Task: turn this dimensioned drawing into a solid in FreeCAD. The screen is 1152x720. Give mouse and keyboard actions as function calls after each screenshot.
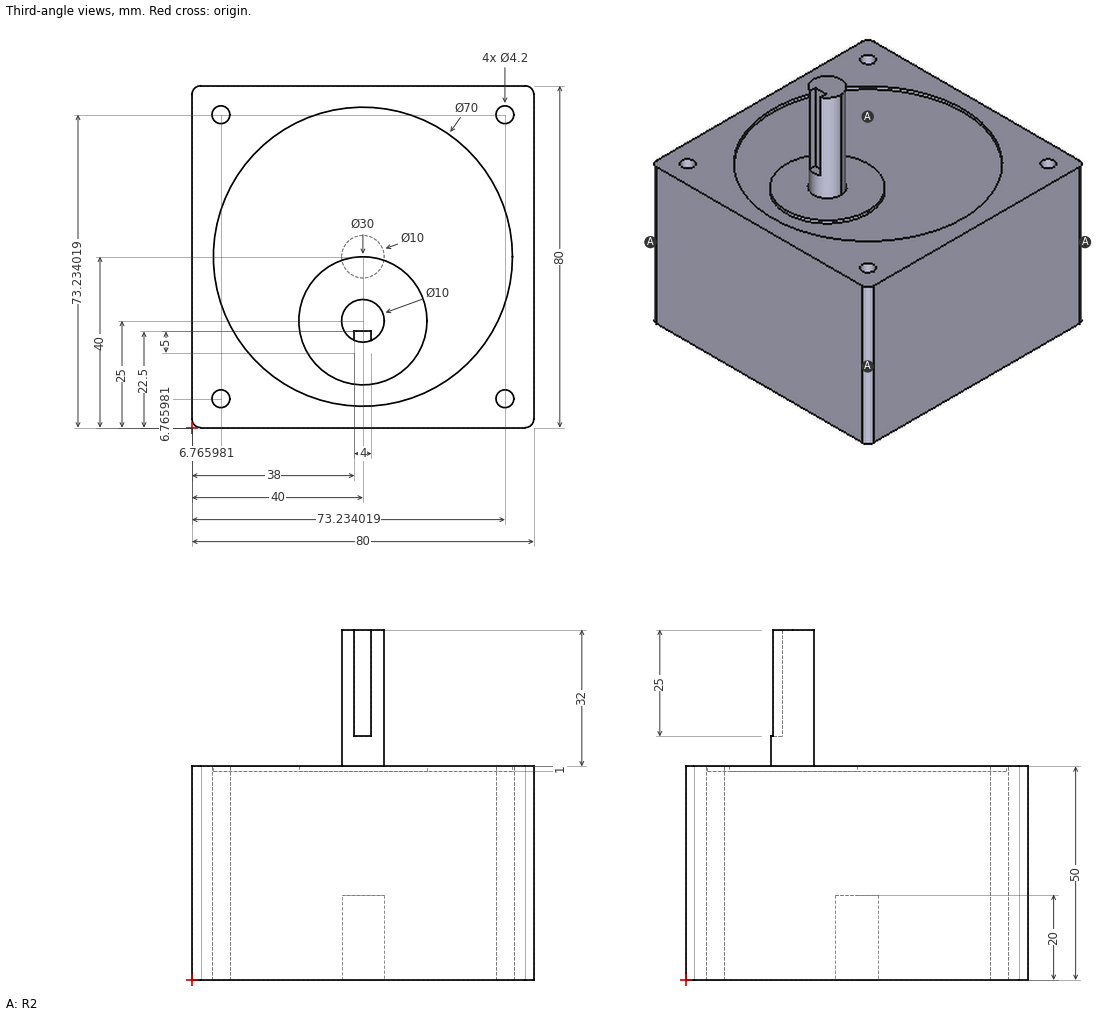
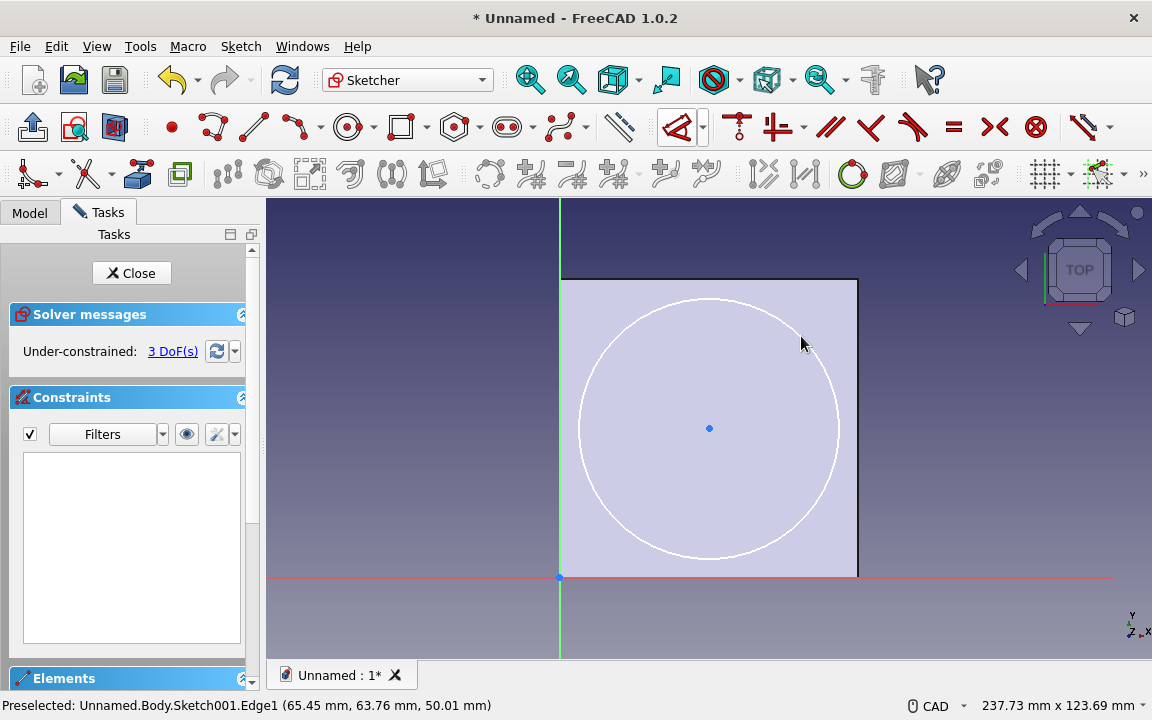
click(801, 337)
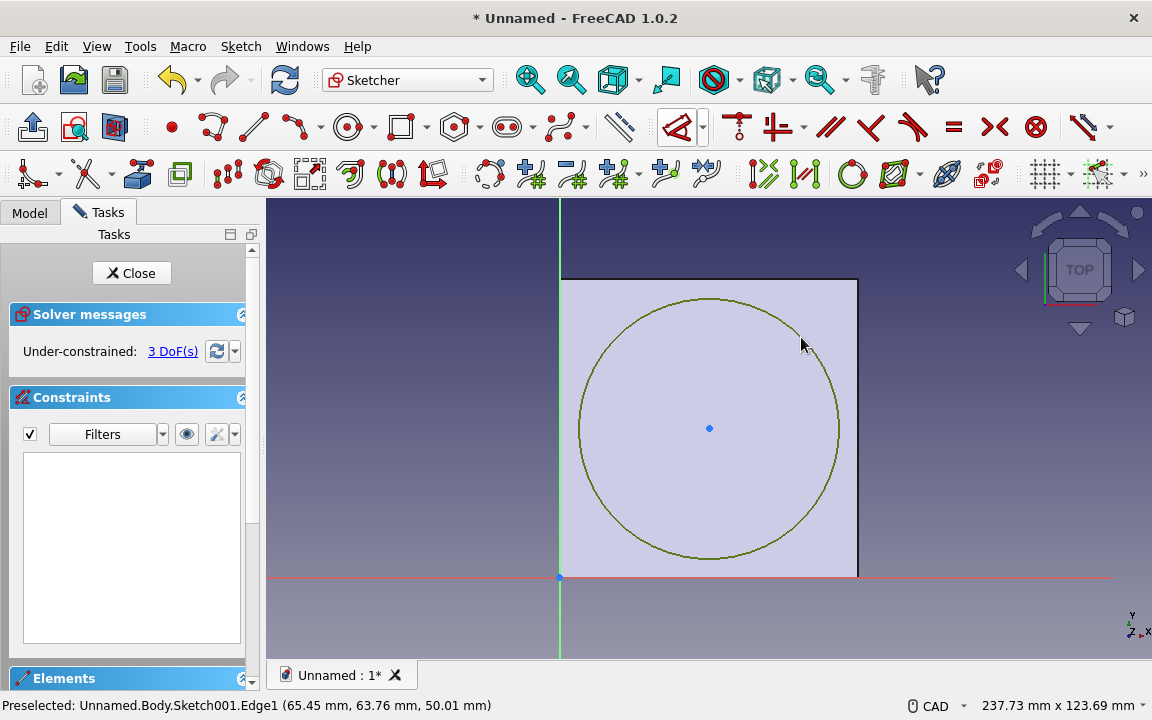
key(k)
key(o)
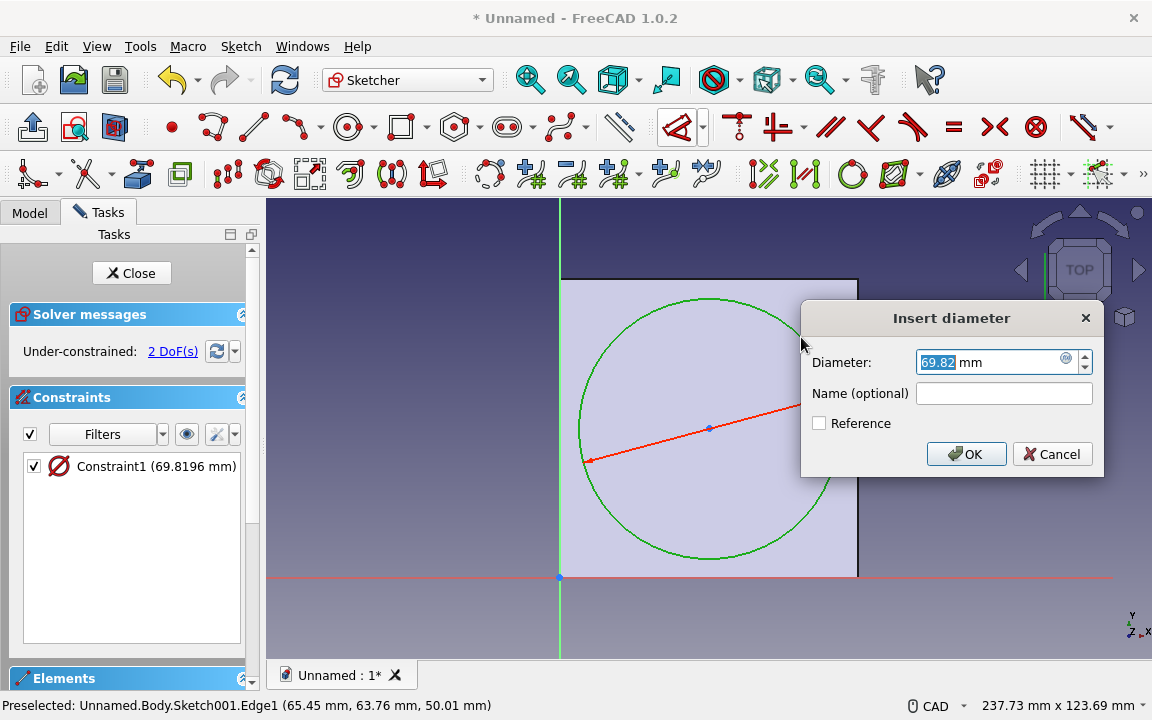
text(70)
key(Return)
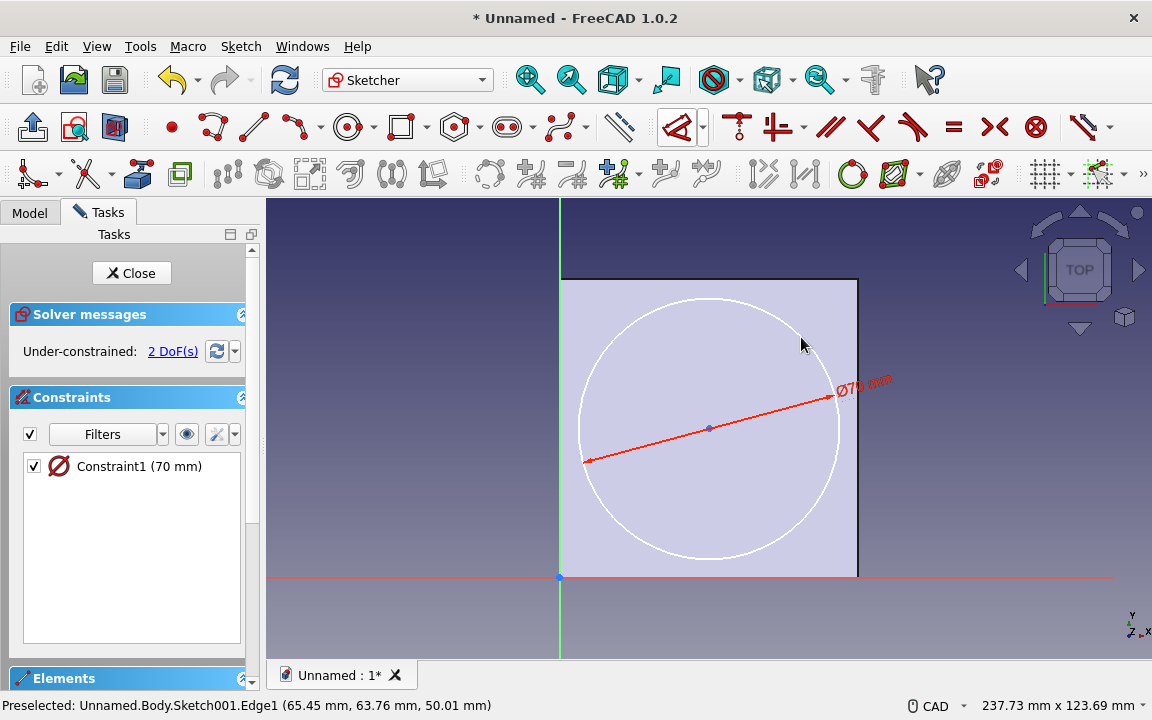
click(709, 429)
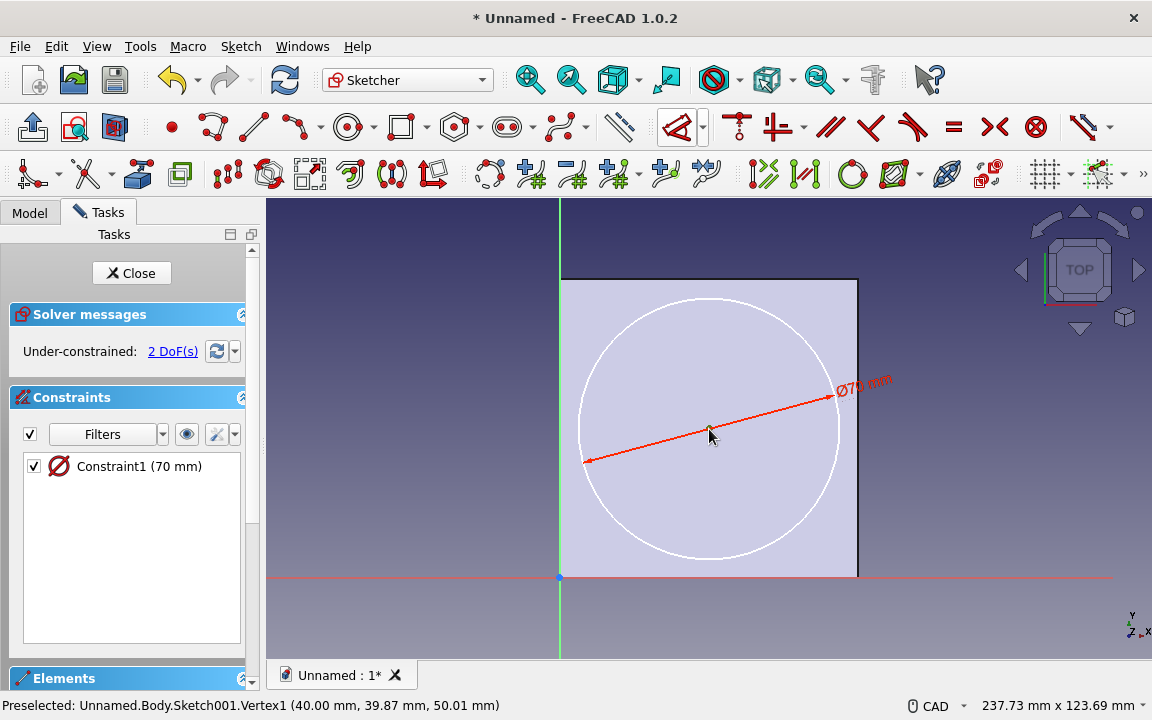
key(l)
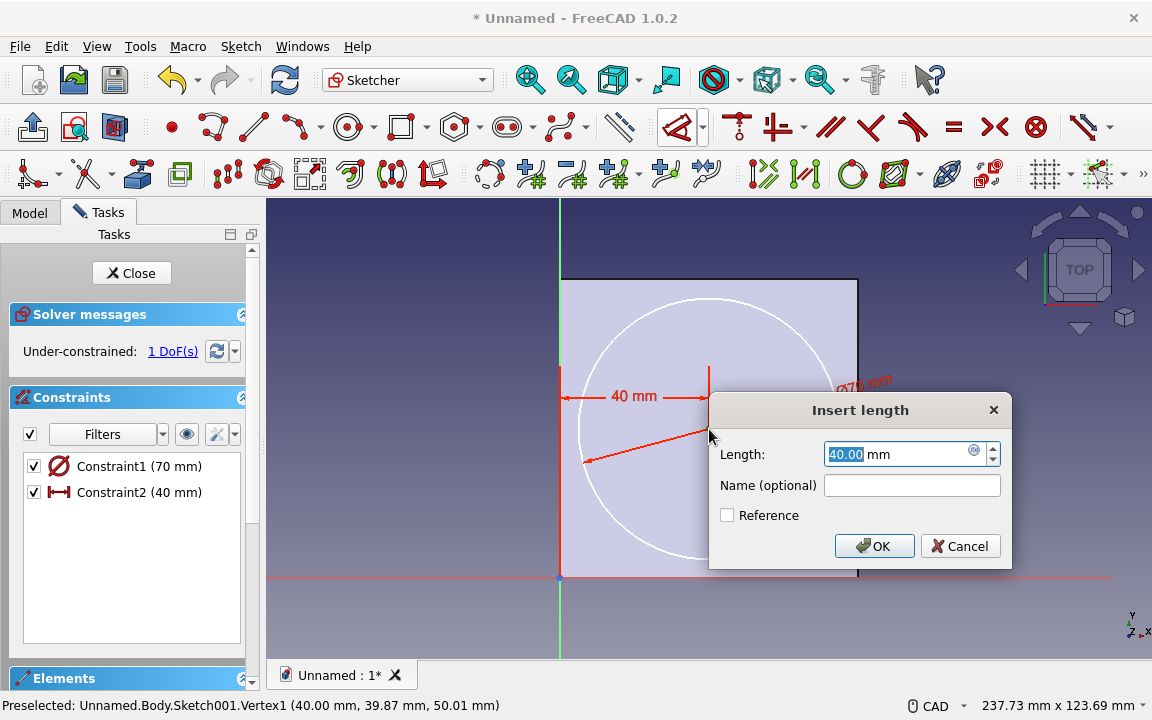
text(40)
key(Return)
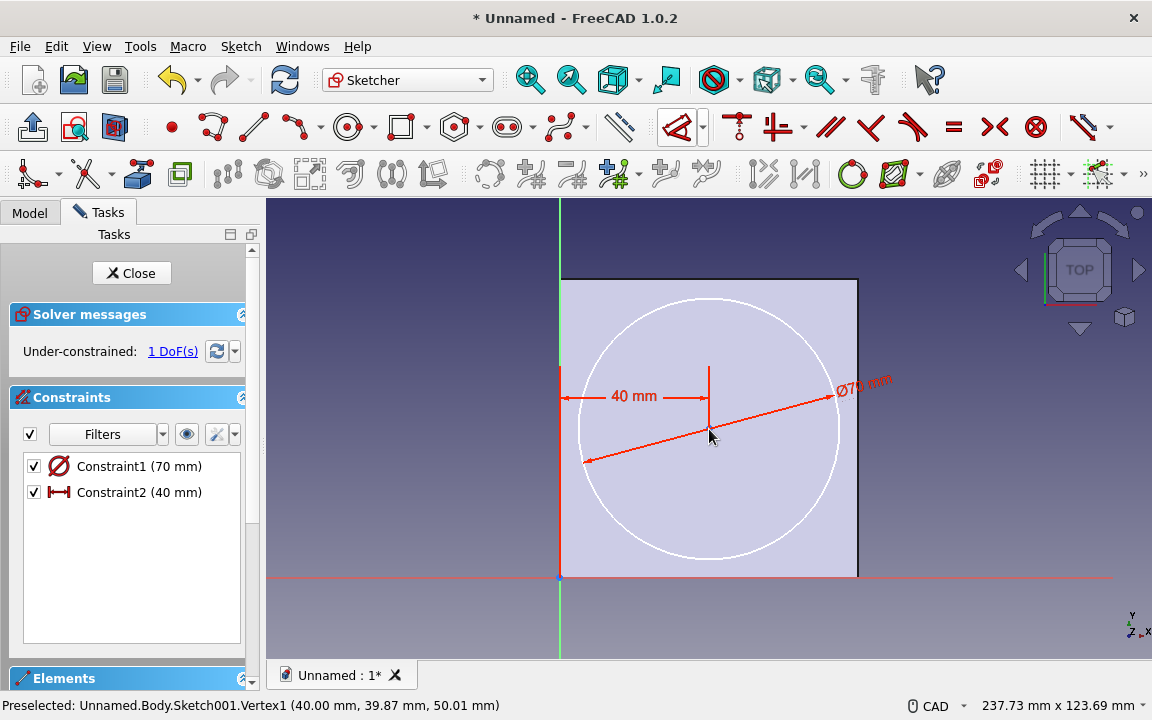
click(709, 429)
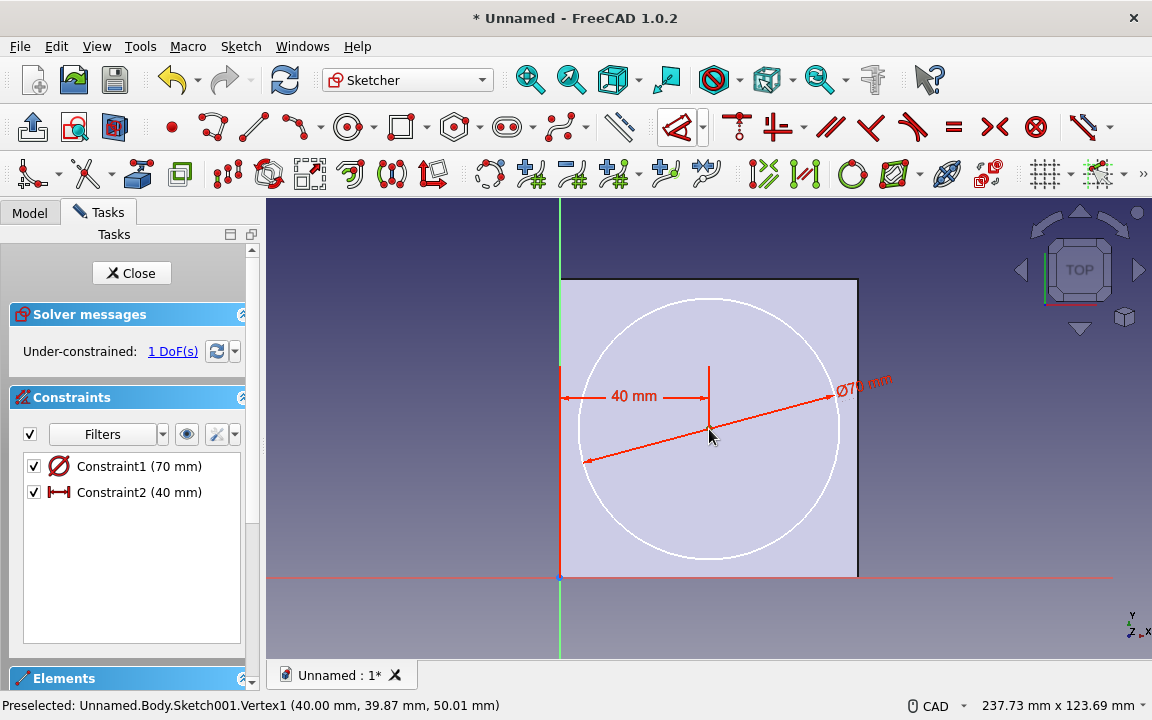
click(702, 128)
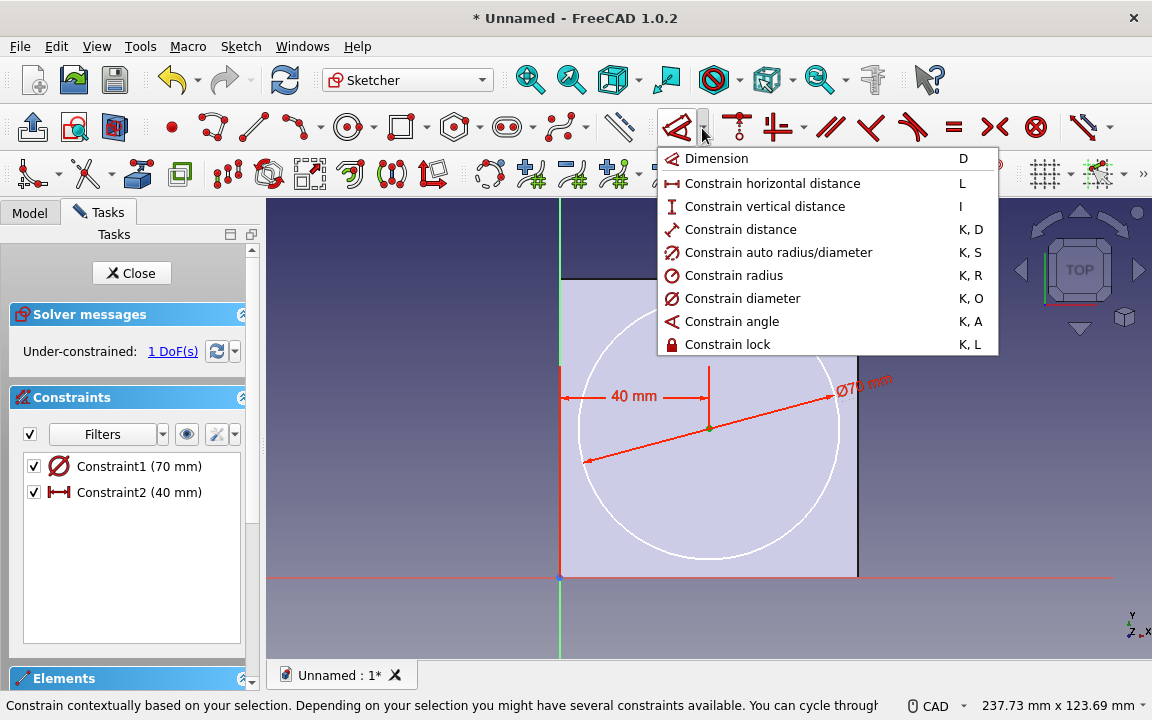
click(828, 206)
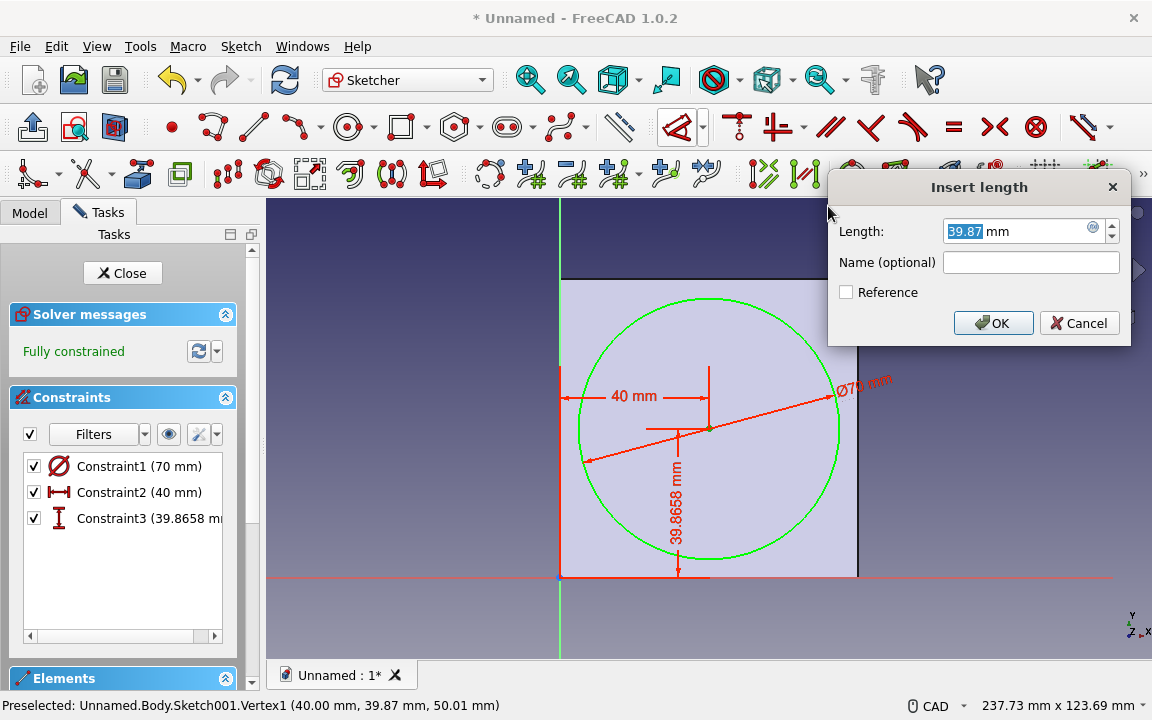
text(40)
key(Return)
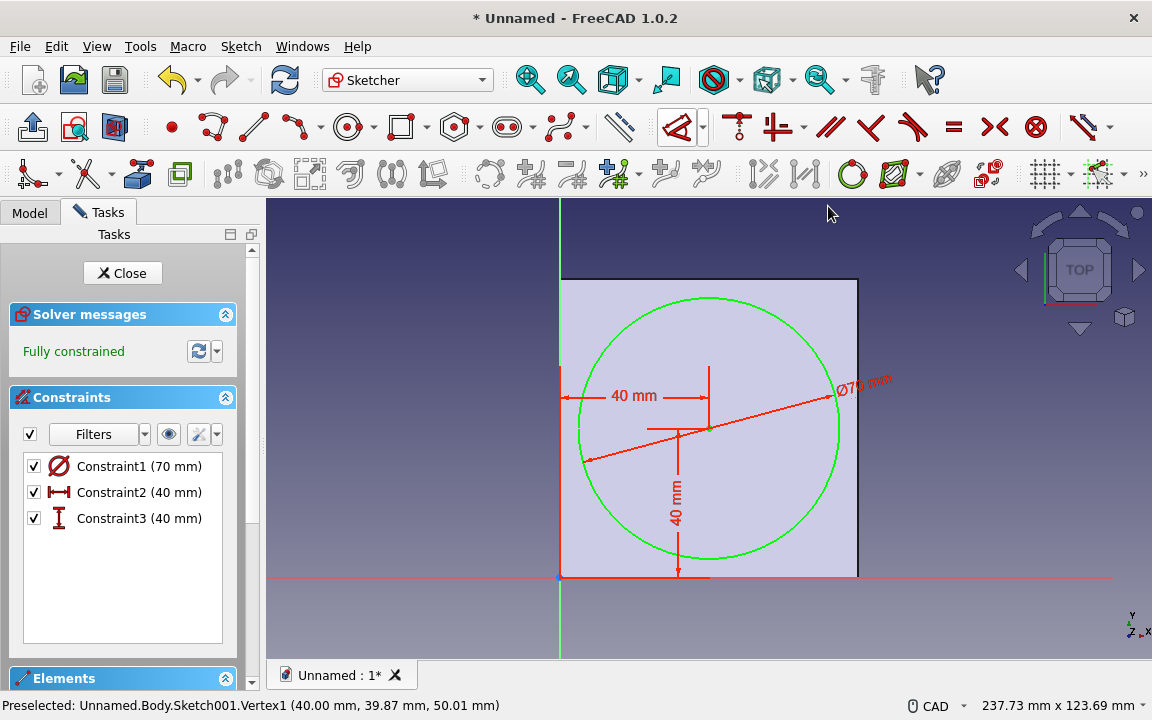
click(123, 273)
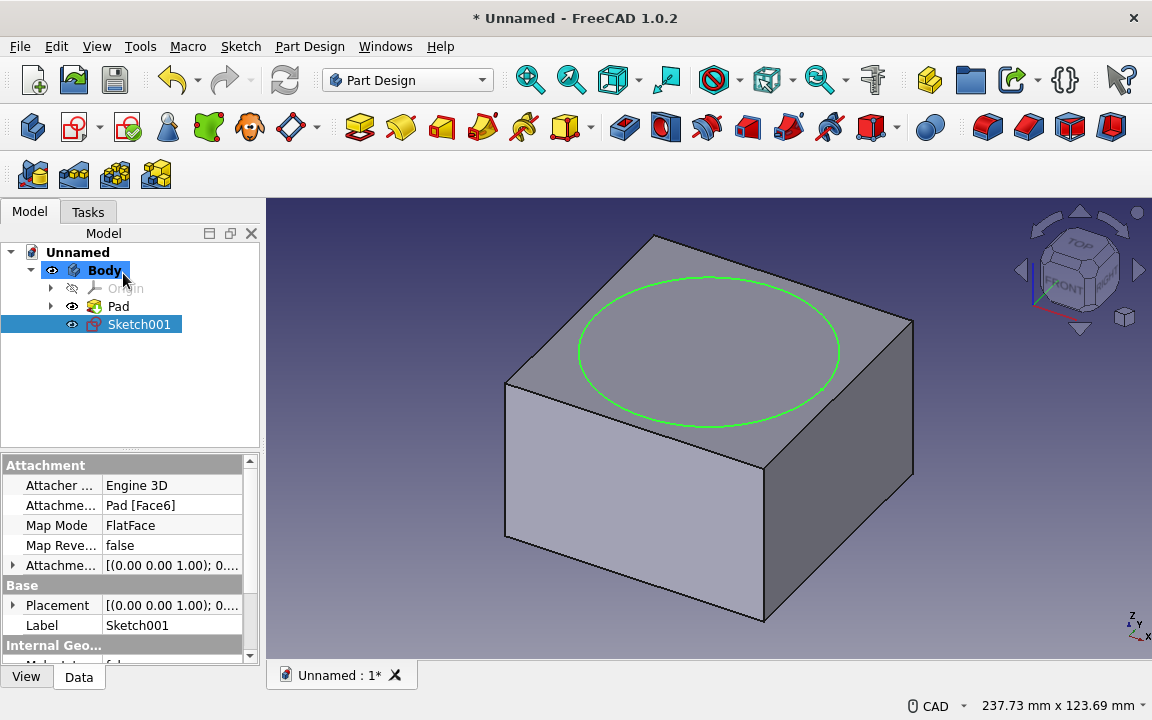
click(625, 128)